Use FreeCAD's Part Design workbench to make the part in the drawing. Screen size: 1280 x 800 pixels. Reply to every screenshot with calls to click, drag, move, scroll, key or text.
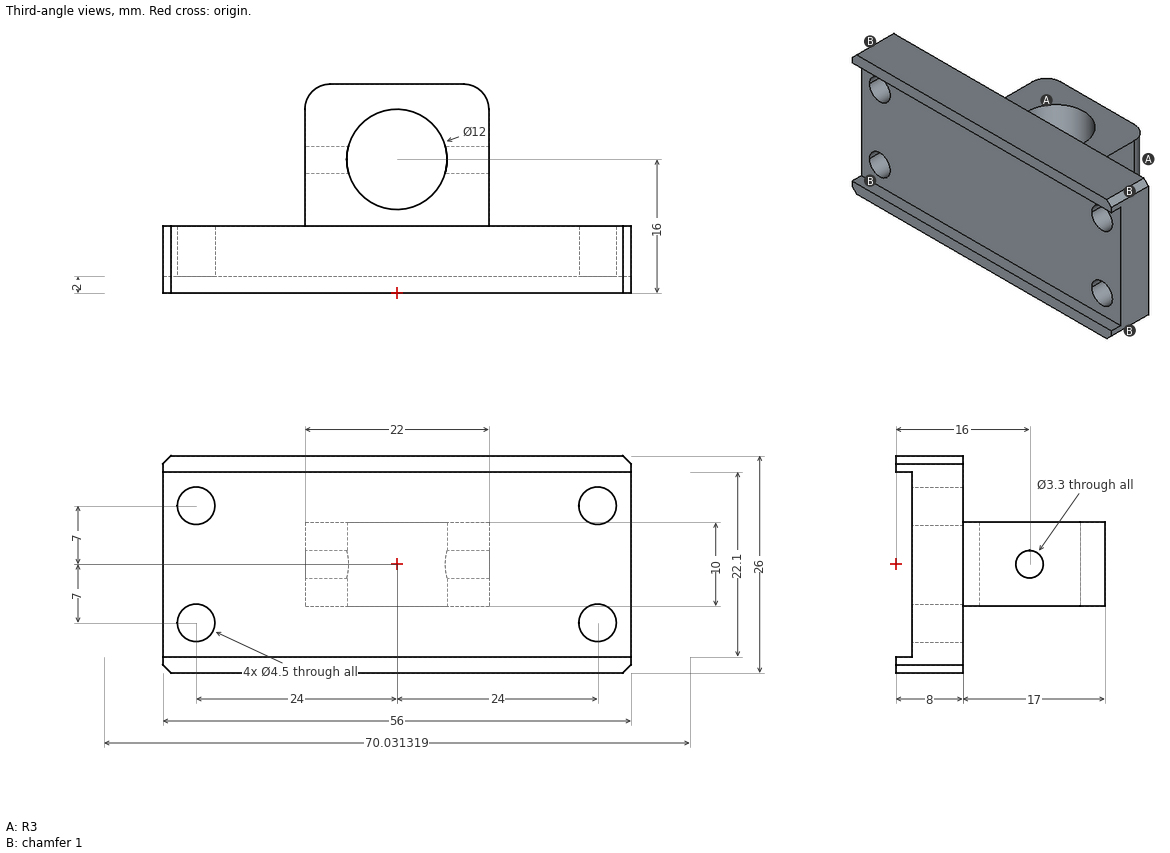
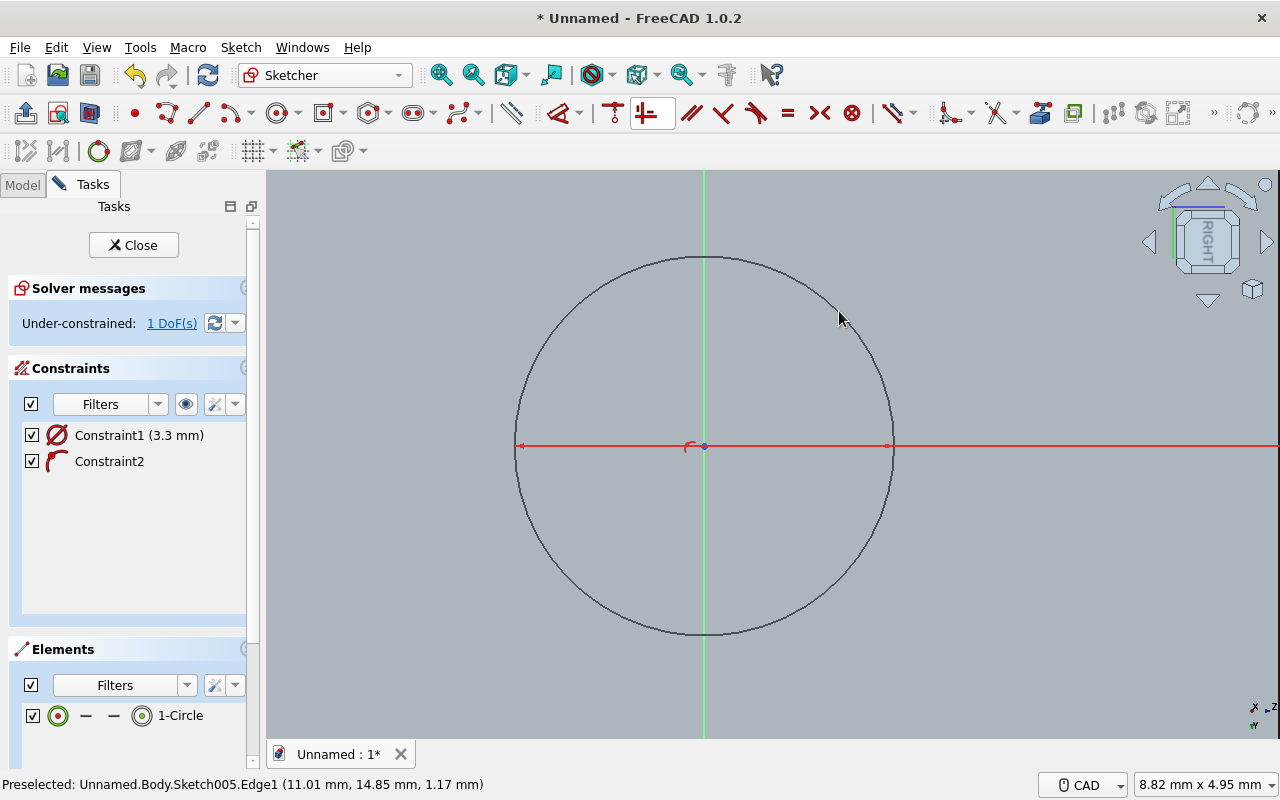
click(558, 114)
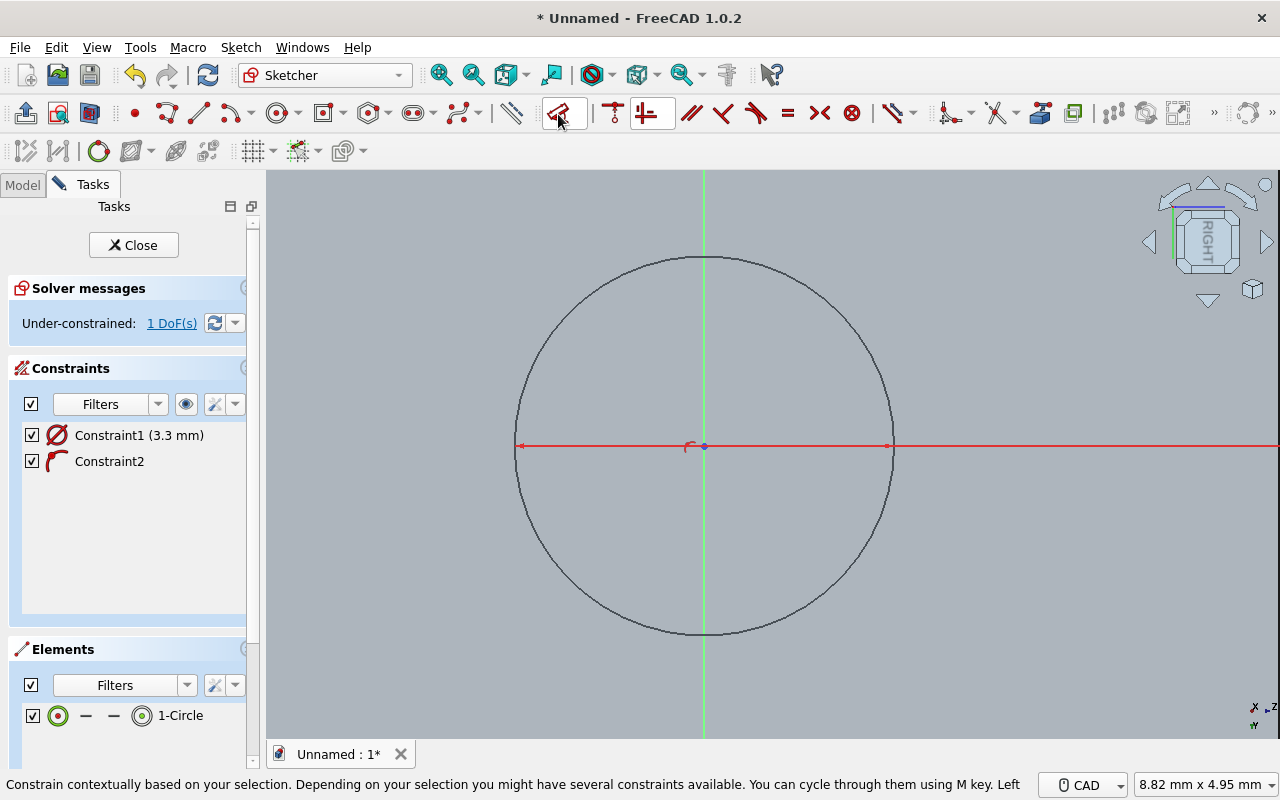
click(704, 446)
click(738, 322)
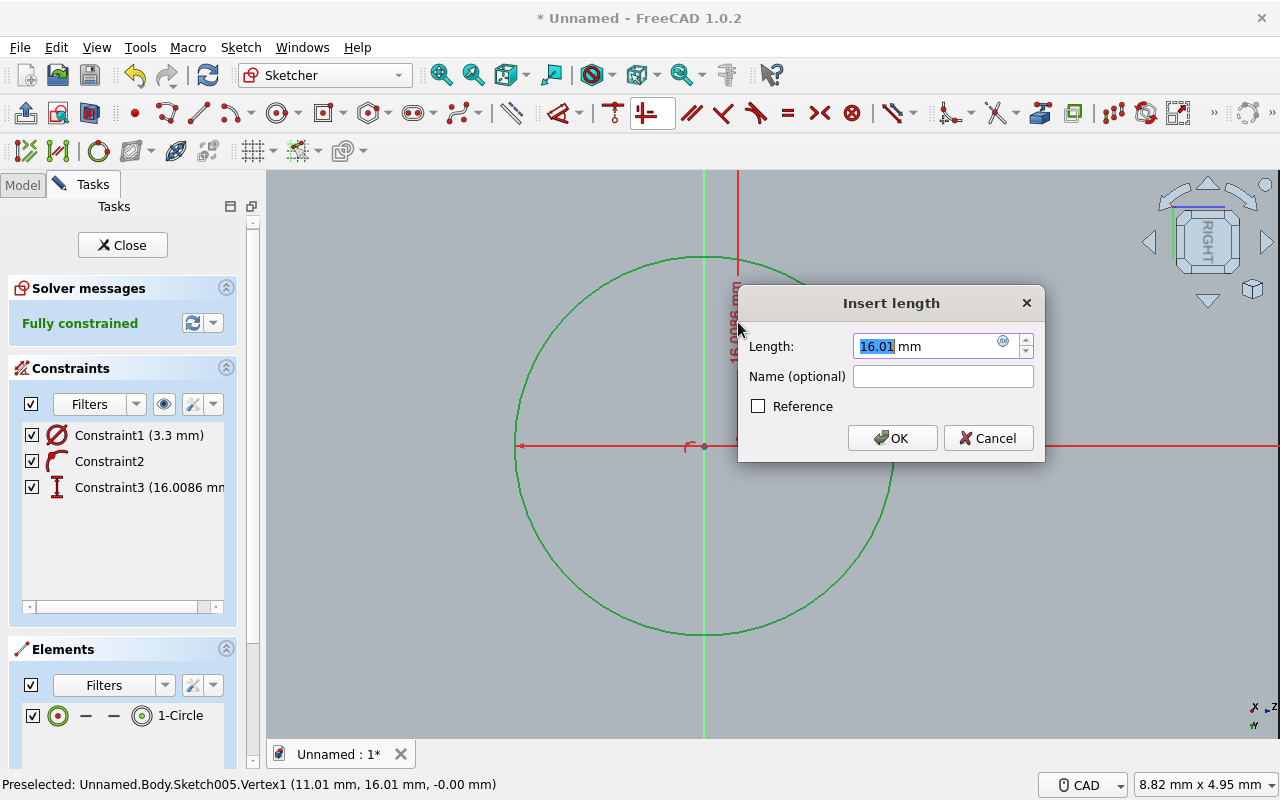
text(16)
key(Return)
key(Escape)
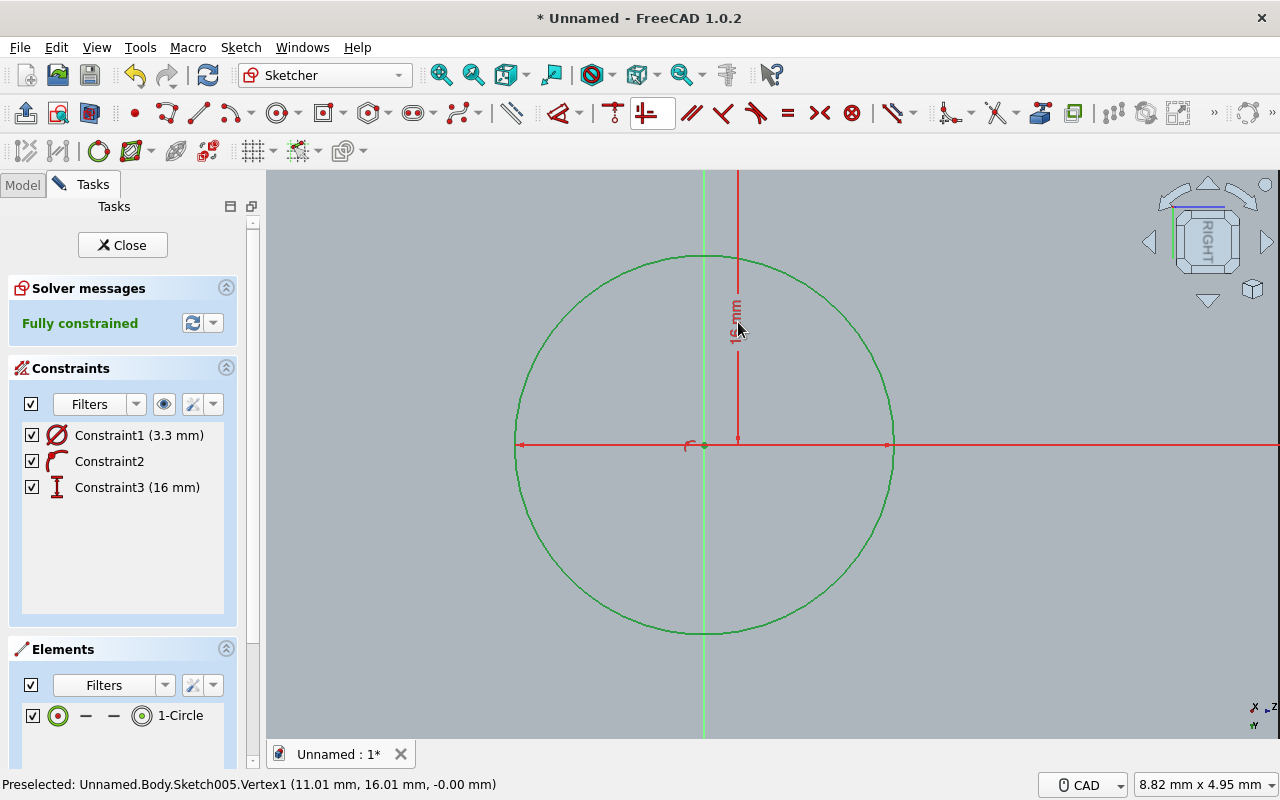
click(123, 245)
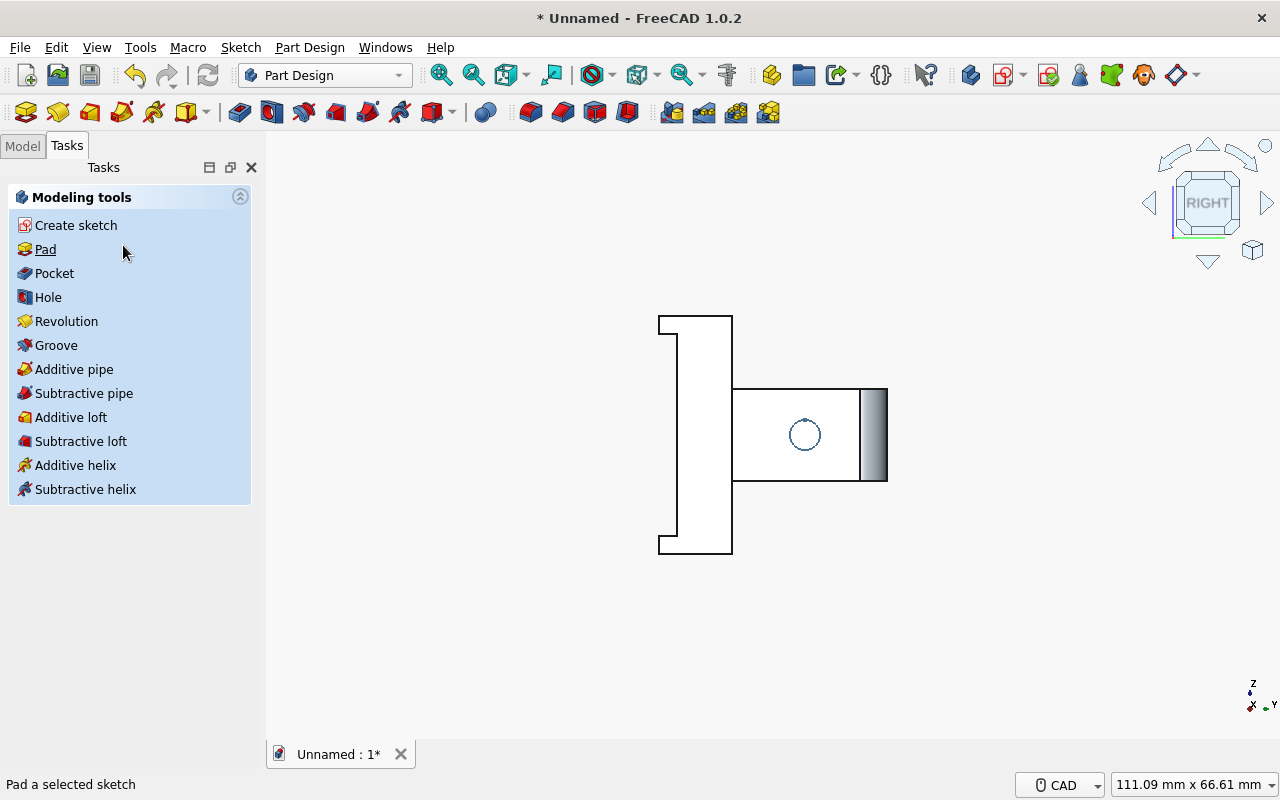
click(272, 112)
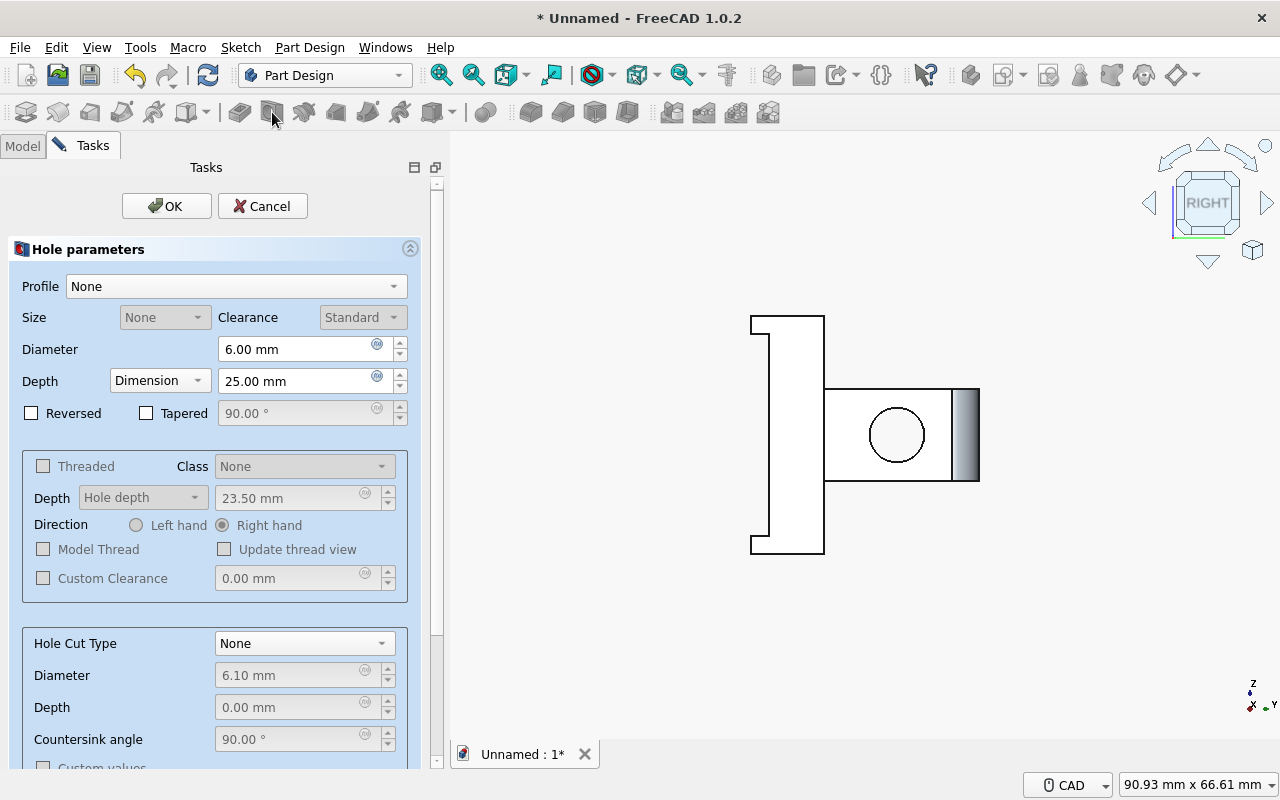
triple_click(305, 349)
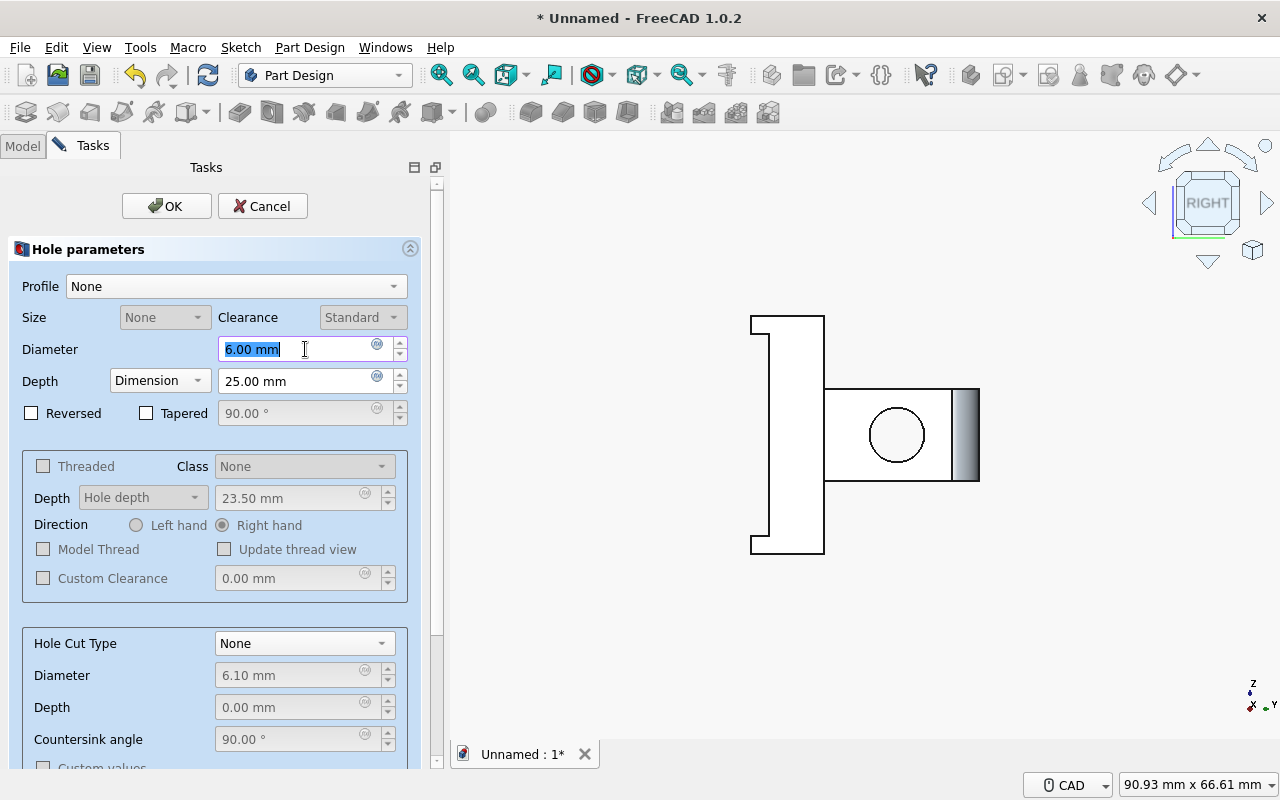
text(3.3)
key(Tab)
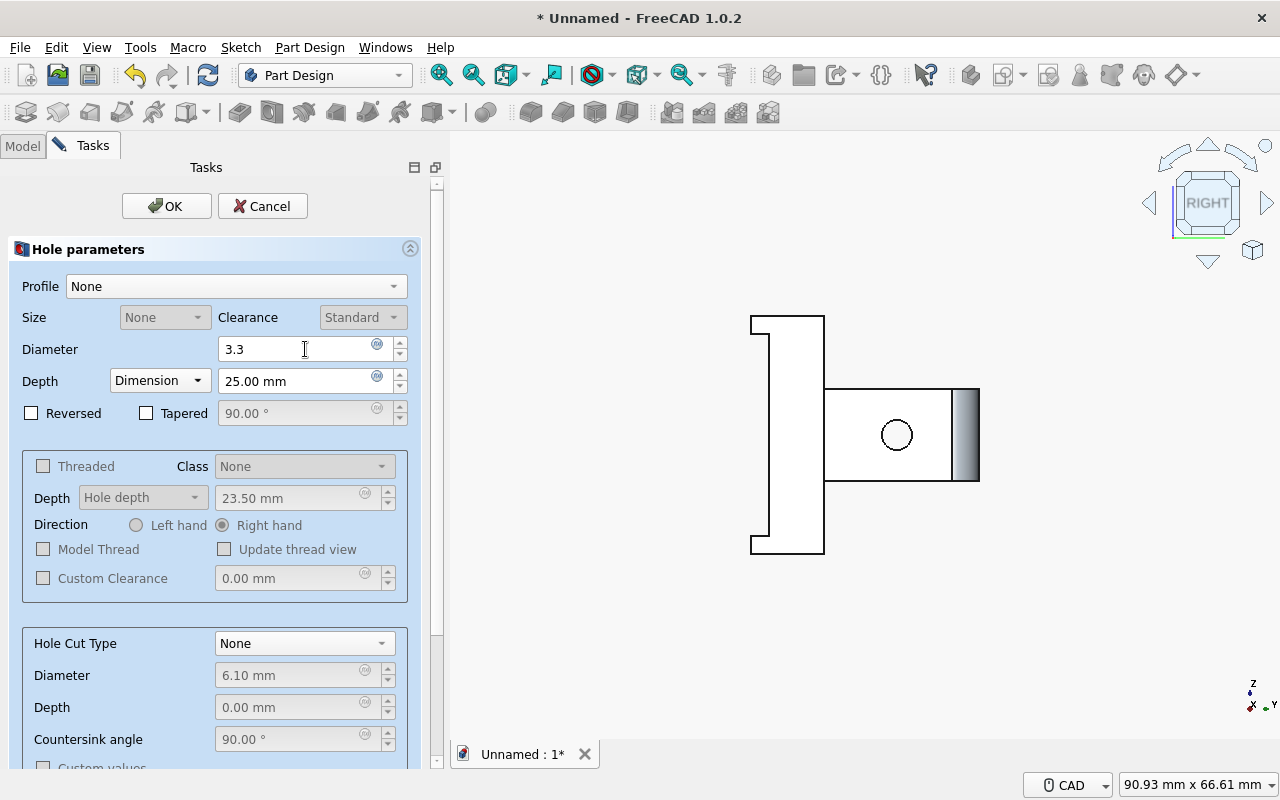
click(161, 380)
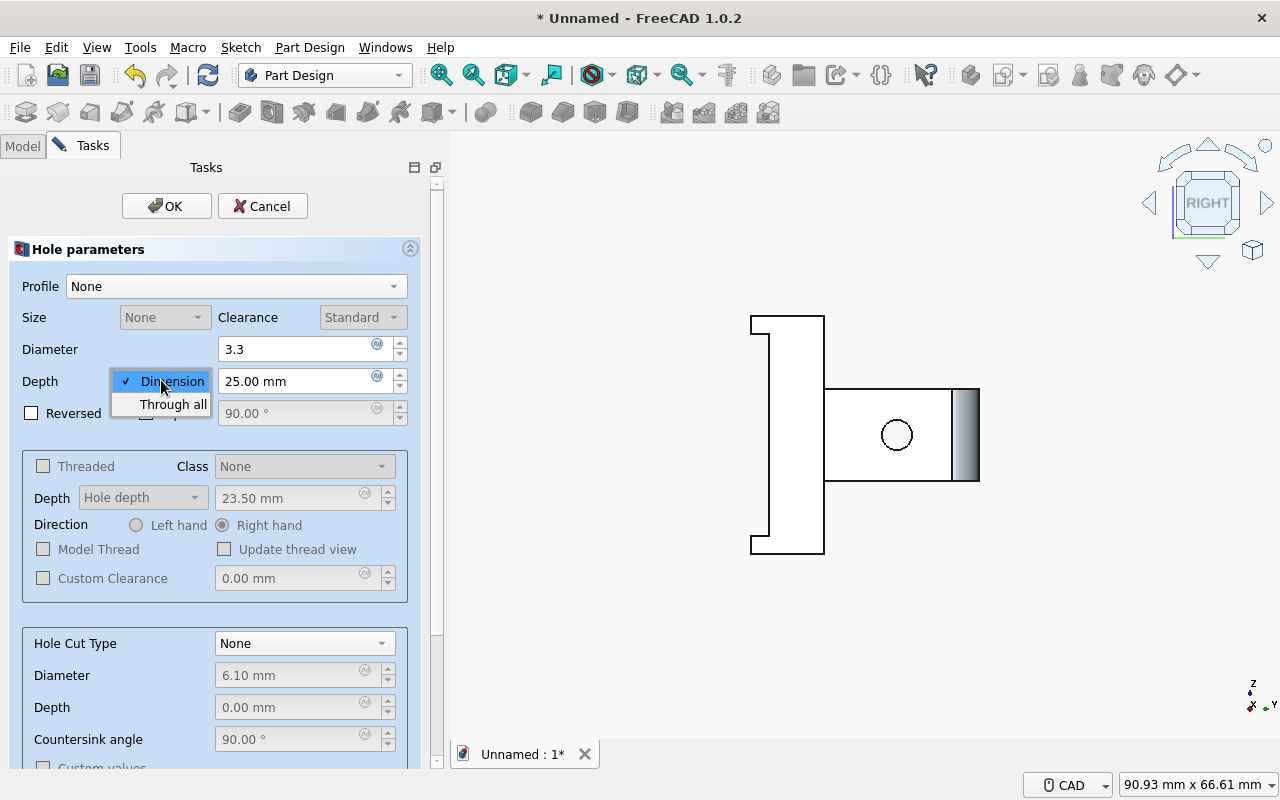
click(160, 404)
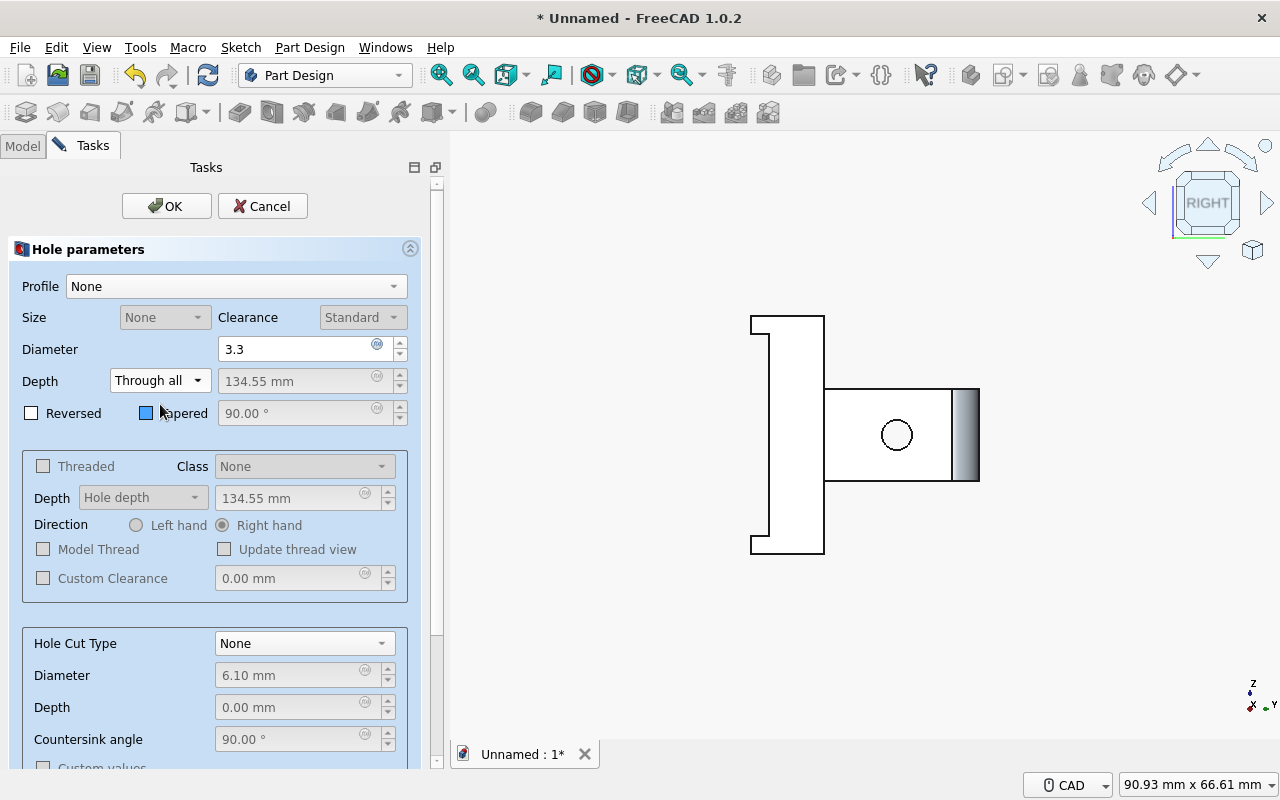
click(167, 206)